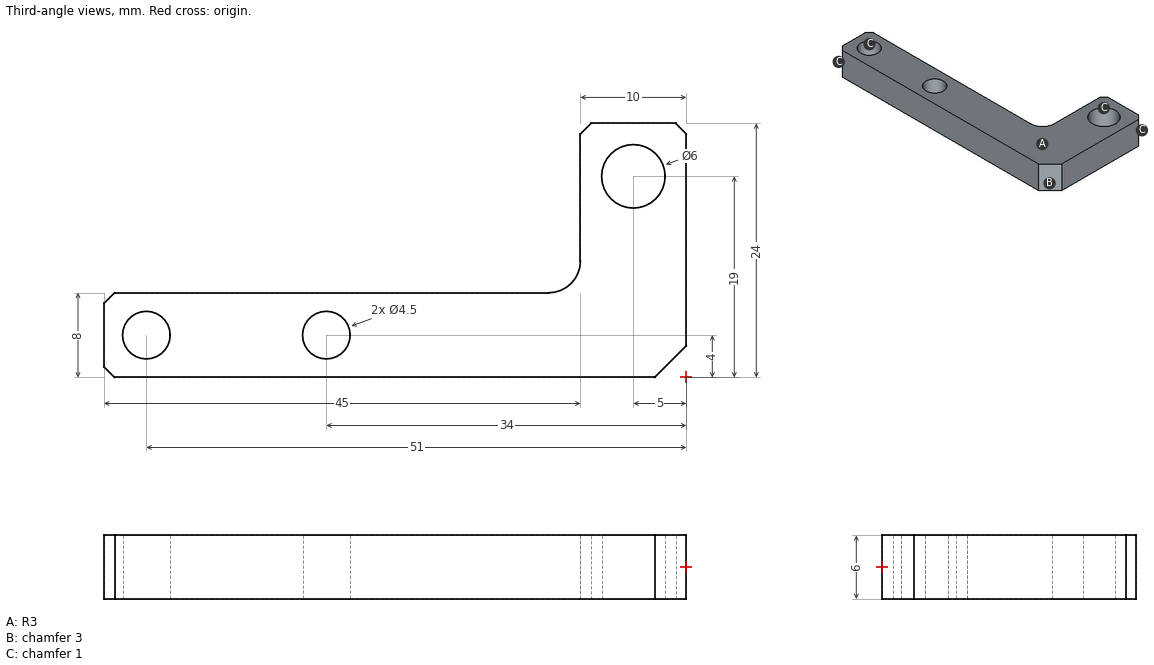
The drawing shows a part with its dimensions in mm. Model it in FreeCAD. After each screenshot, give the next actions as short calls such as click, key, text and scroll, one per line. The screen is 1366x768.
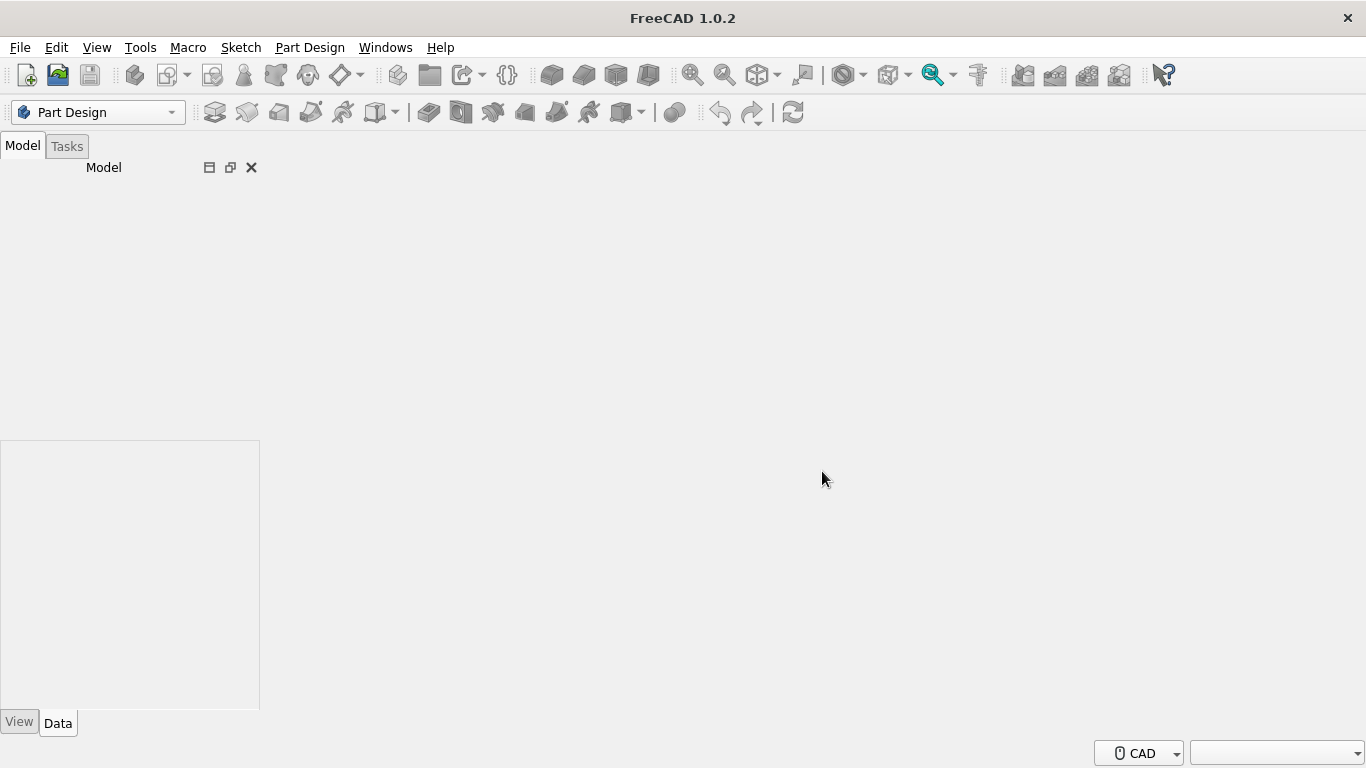
key(ctrl+n)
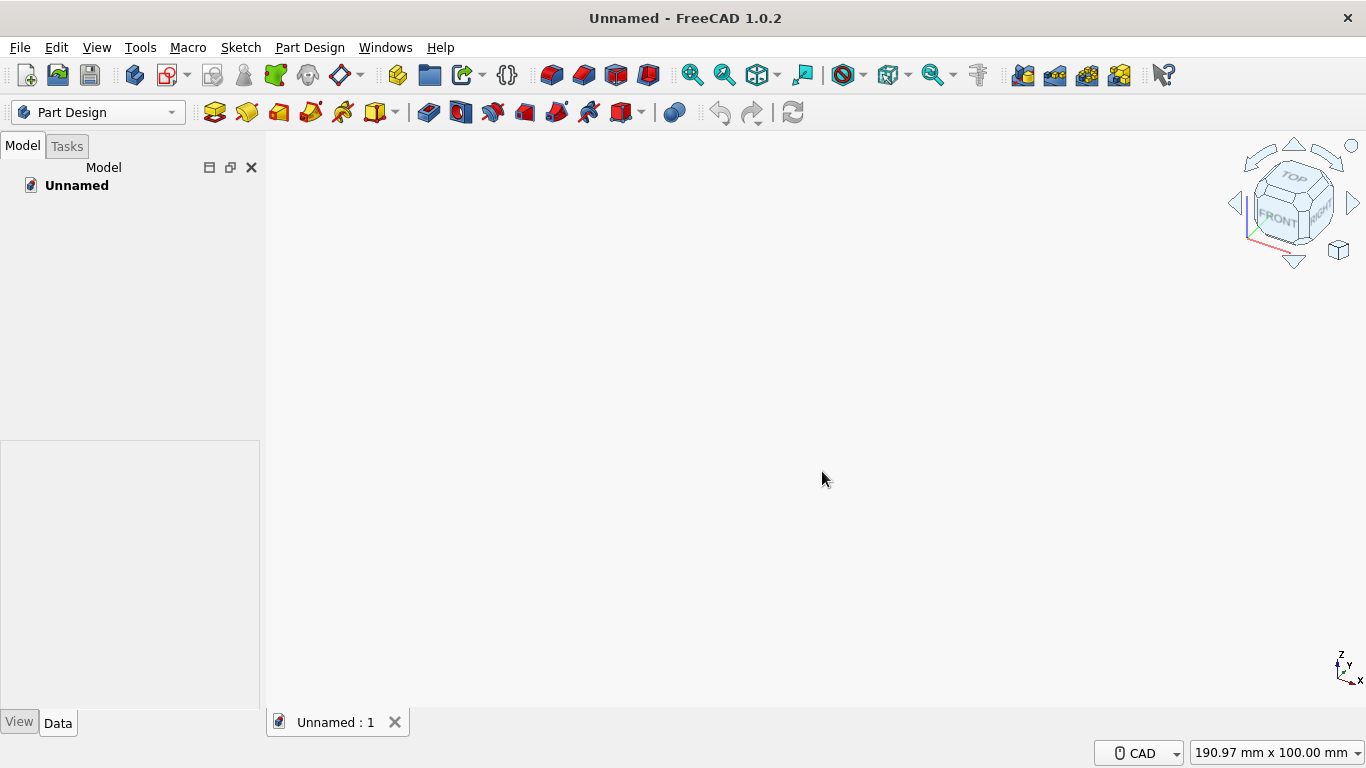
click(168, 76)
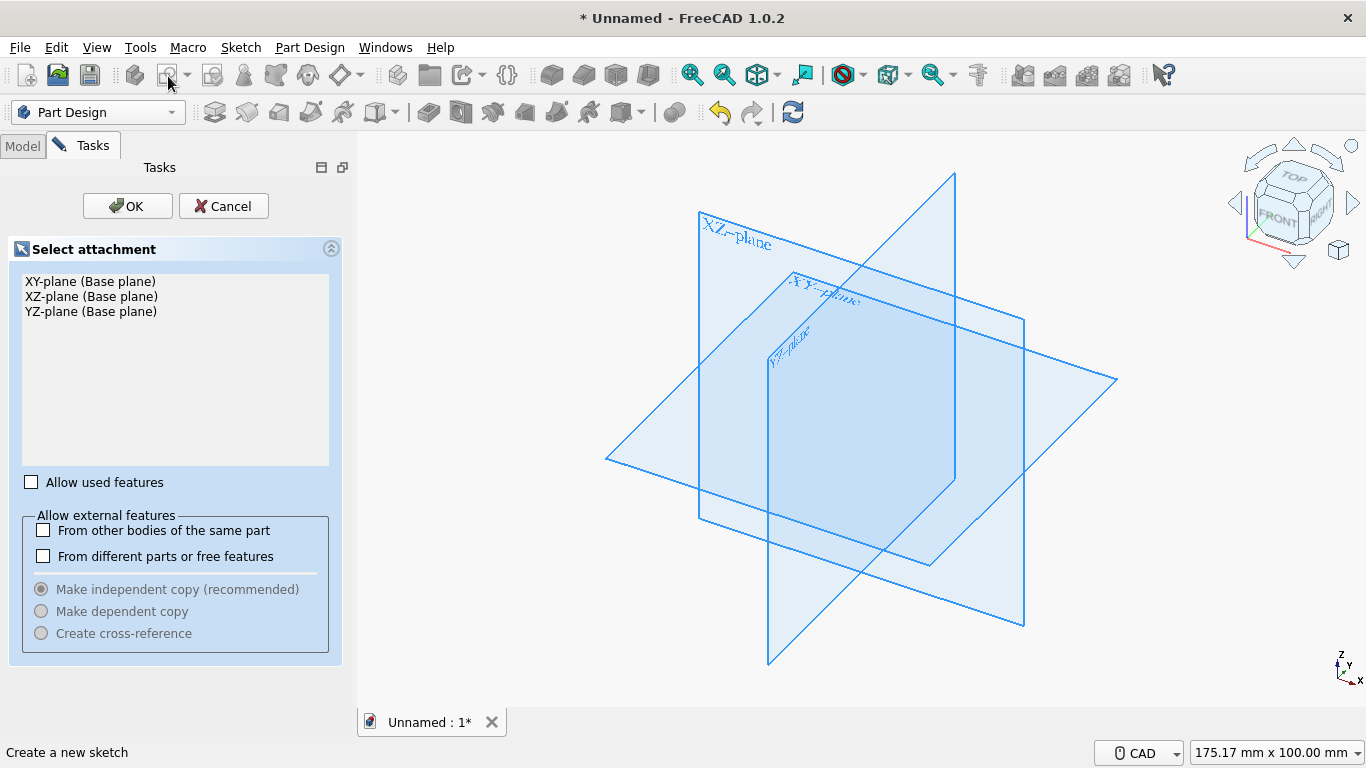
click(82, 282)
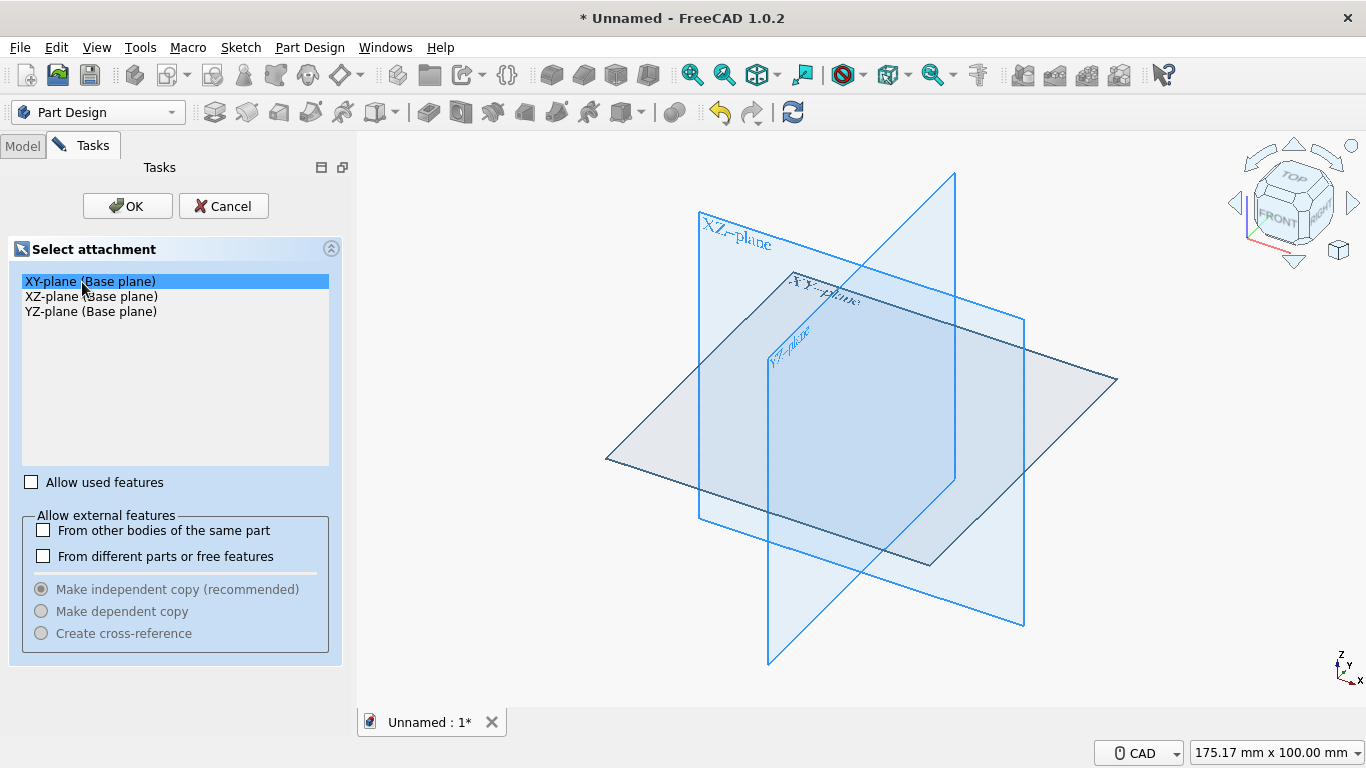
click(128, 206)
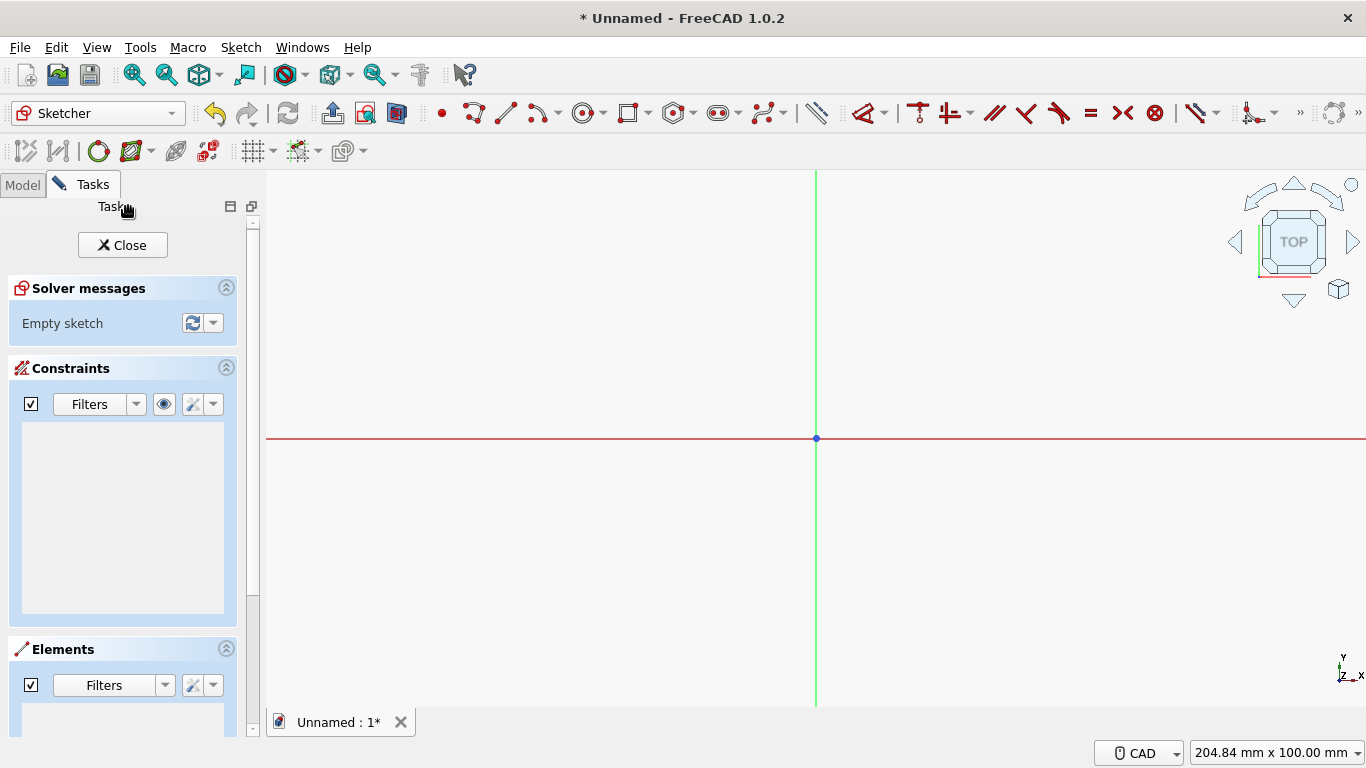
scroll(604, 321, up, 4)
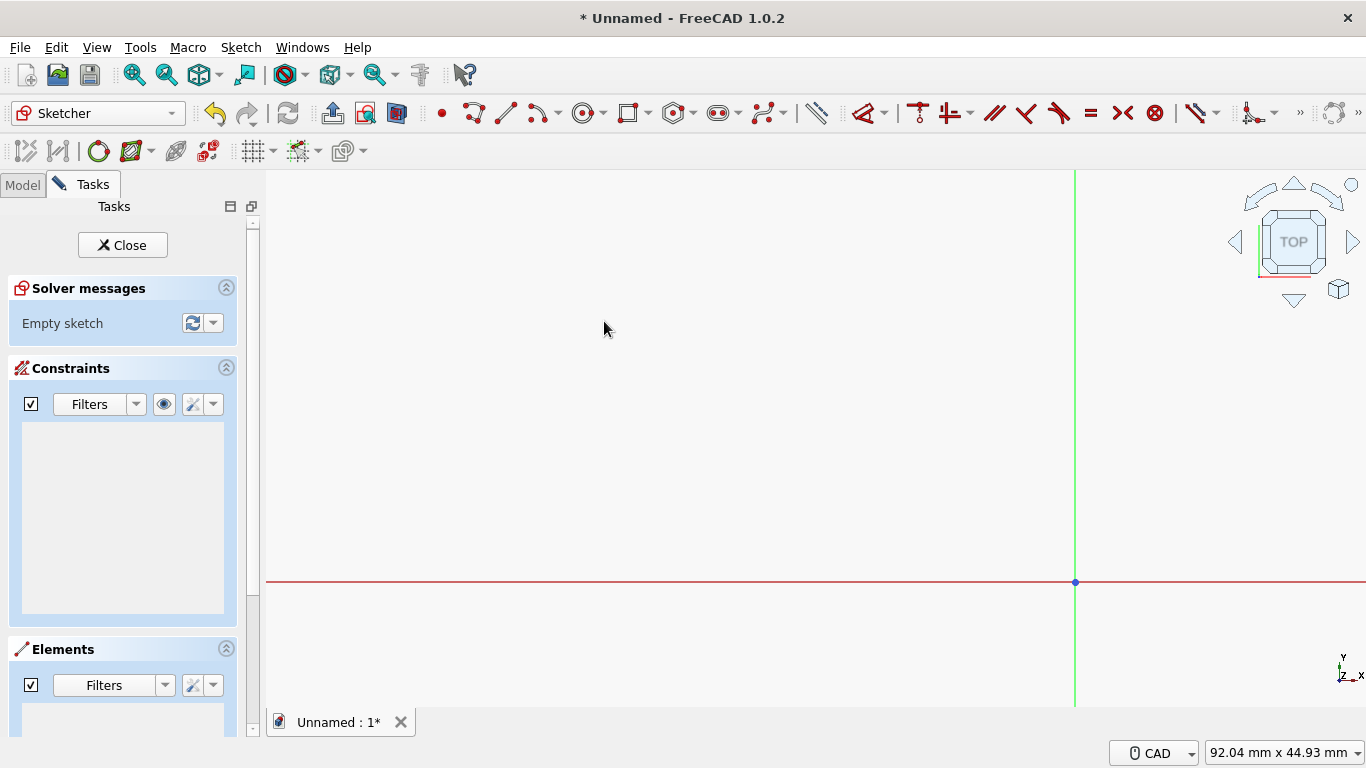
click(474, 114)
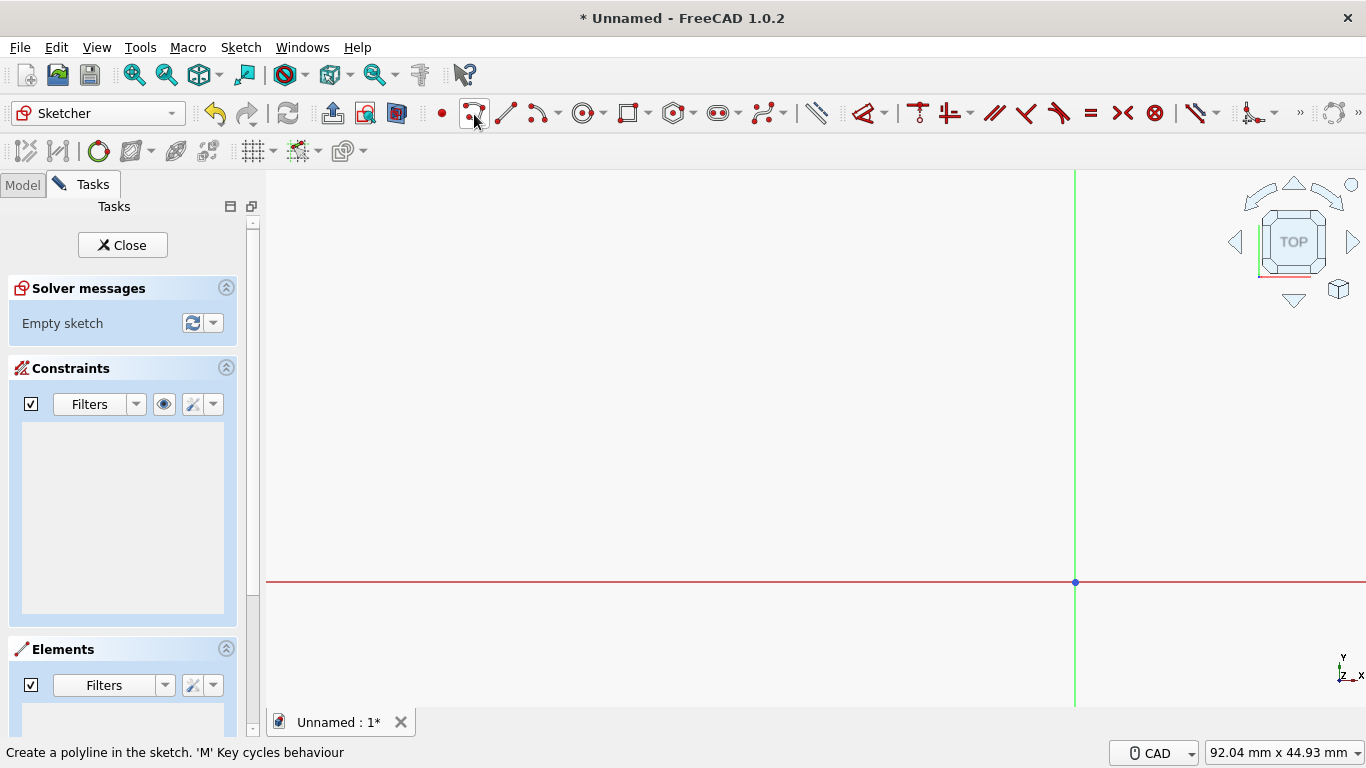
click(1075, 582)
click(1066, 295)
click(956, 295)
click(956, 487)
click(418, 487)
click(418, 573)
click(1075, 582)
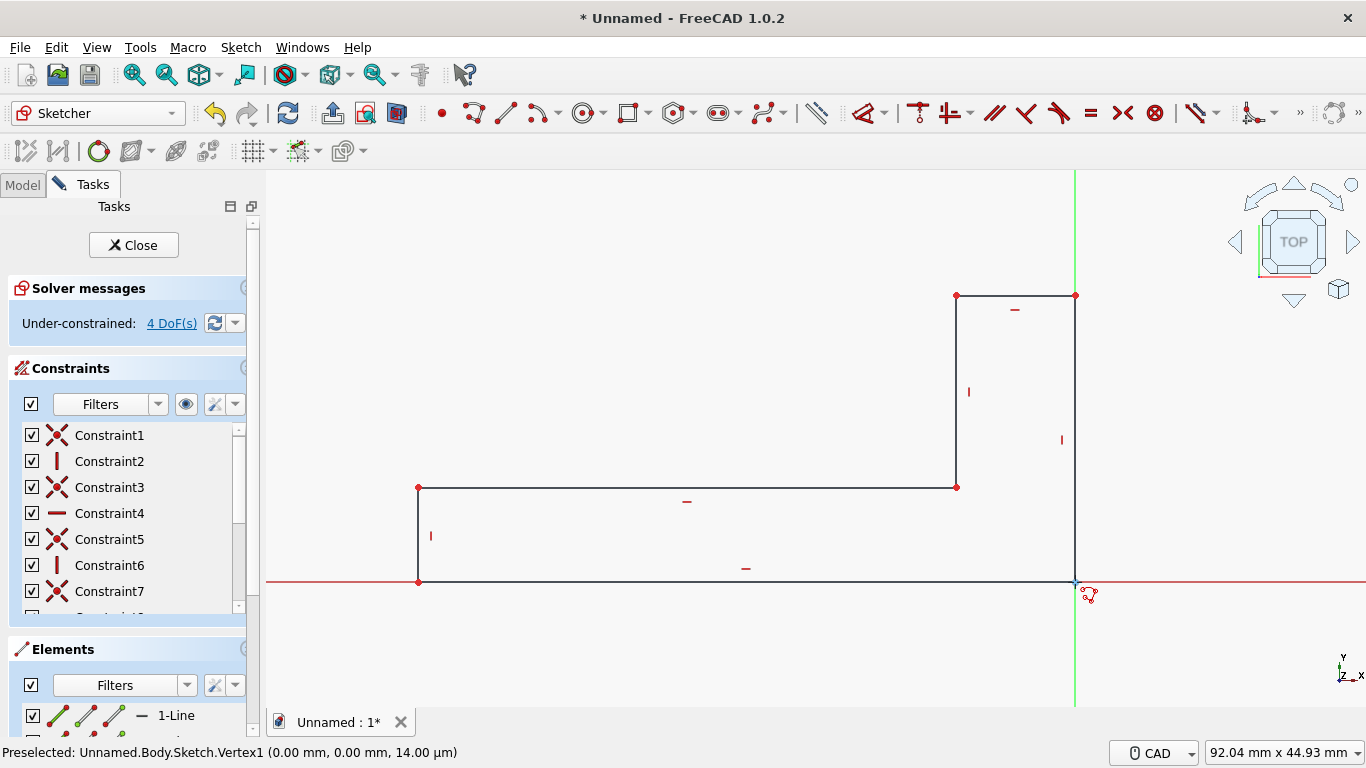
key(g)
key(c)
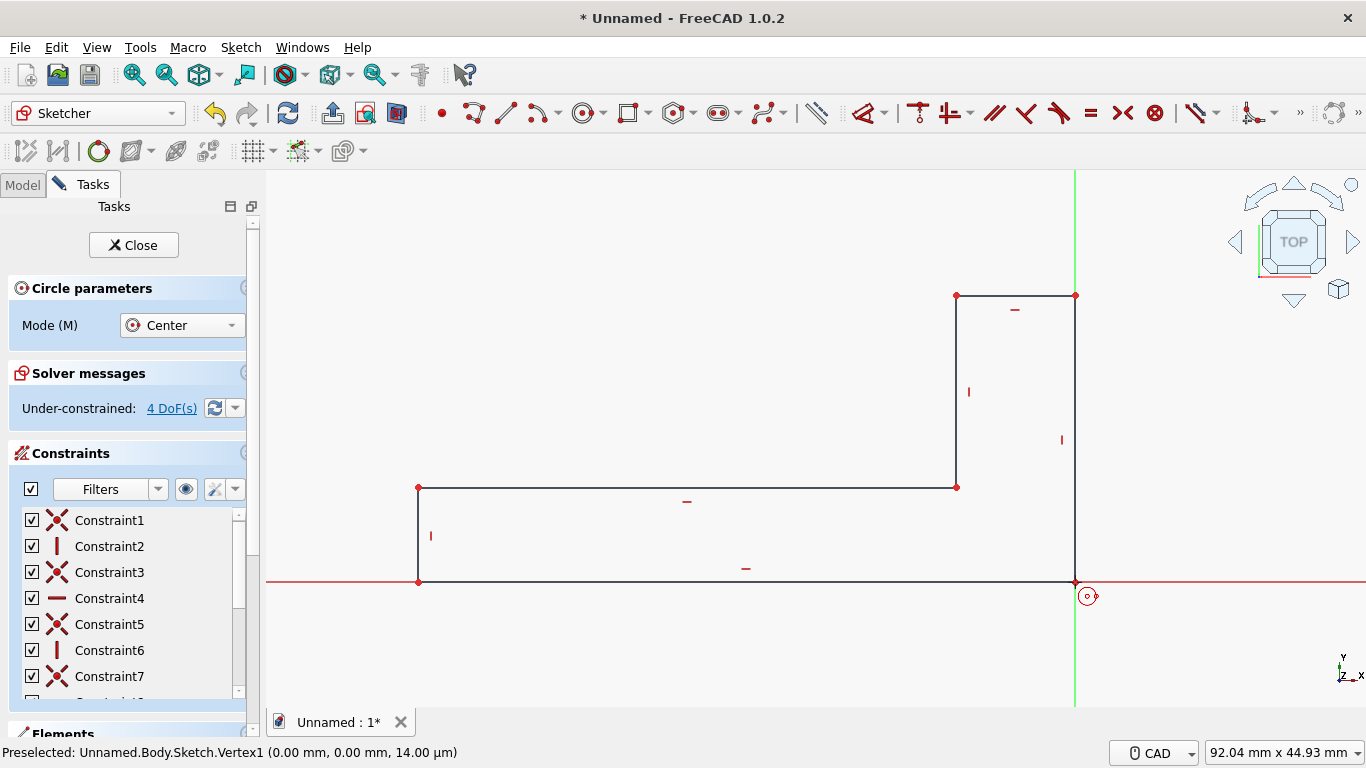
click(669, 534)
click(688, 515)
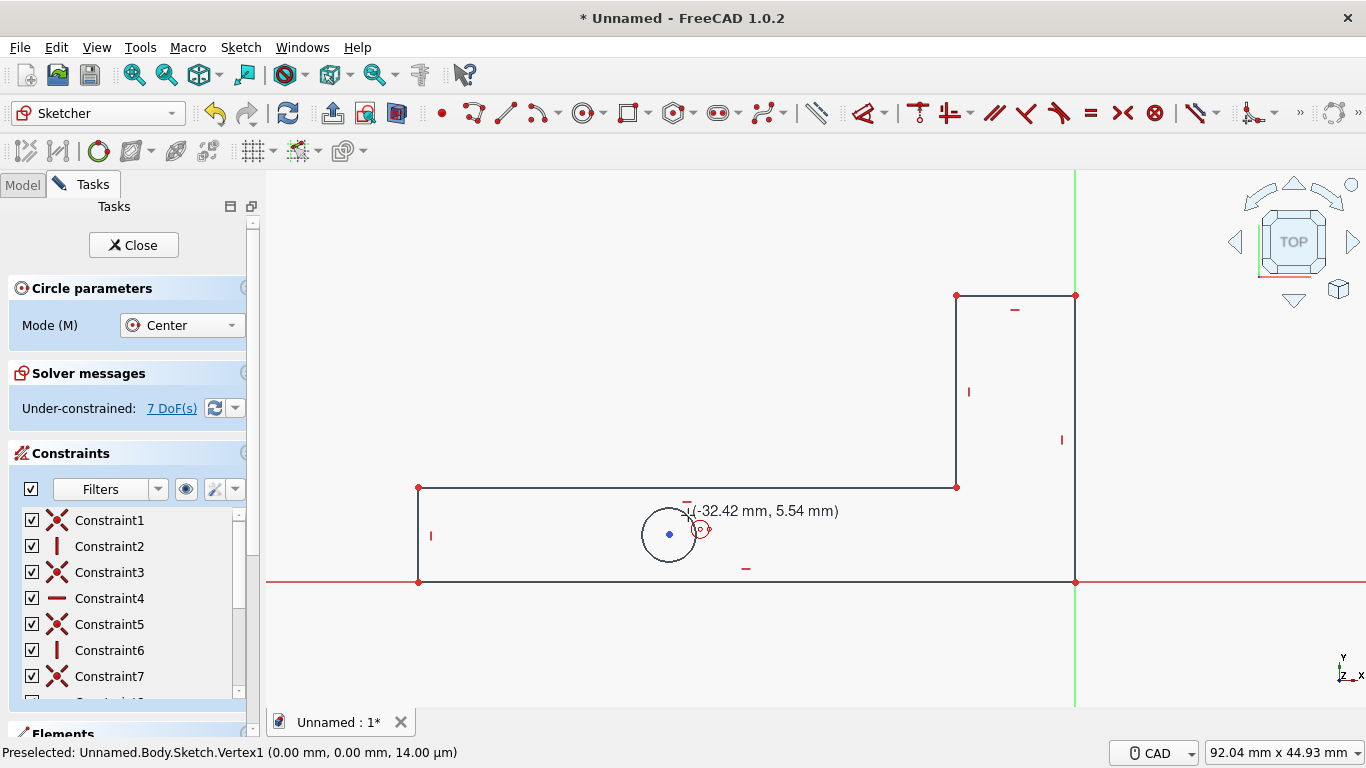
click(466, 534)
click(485, 515)